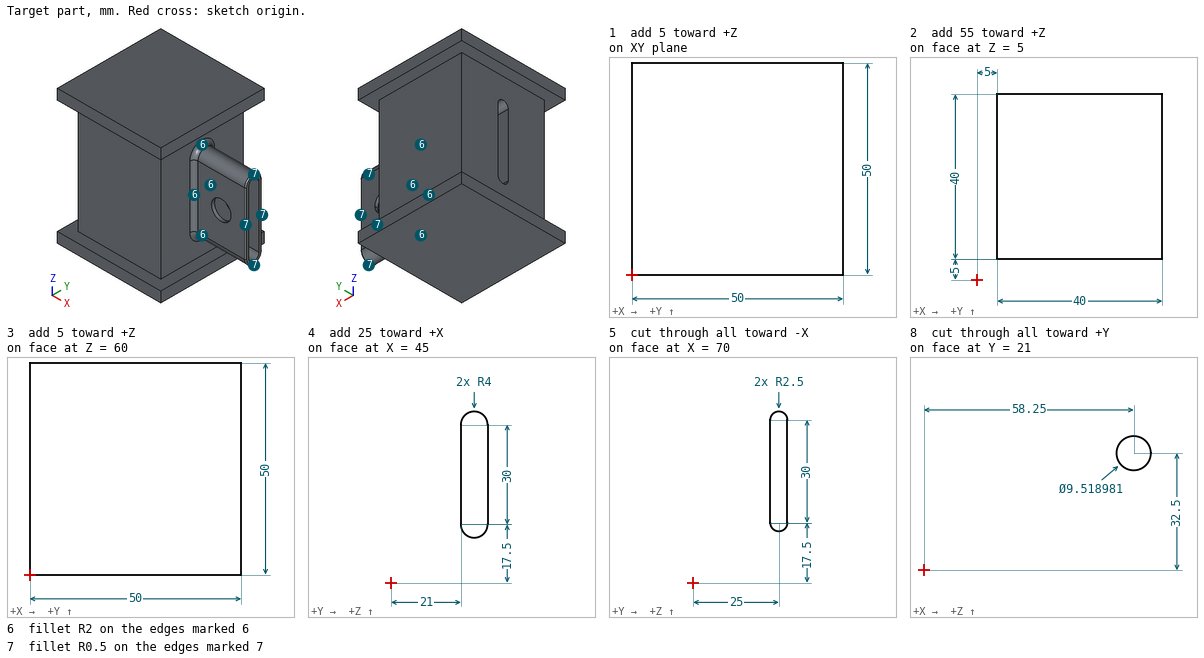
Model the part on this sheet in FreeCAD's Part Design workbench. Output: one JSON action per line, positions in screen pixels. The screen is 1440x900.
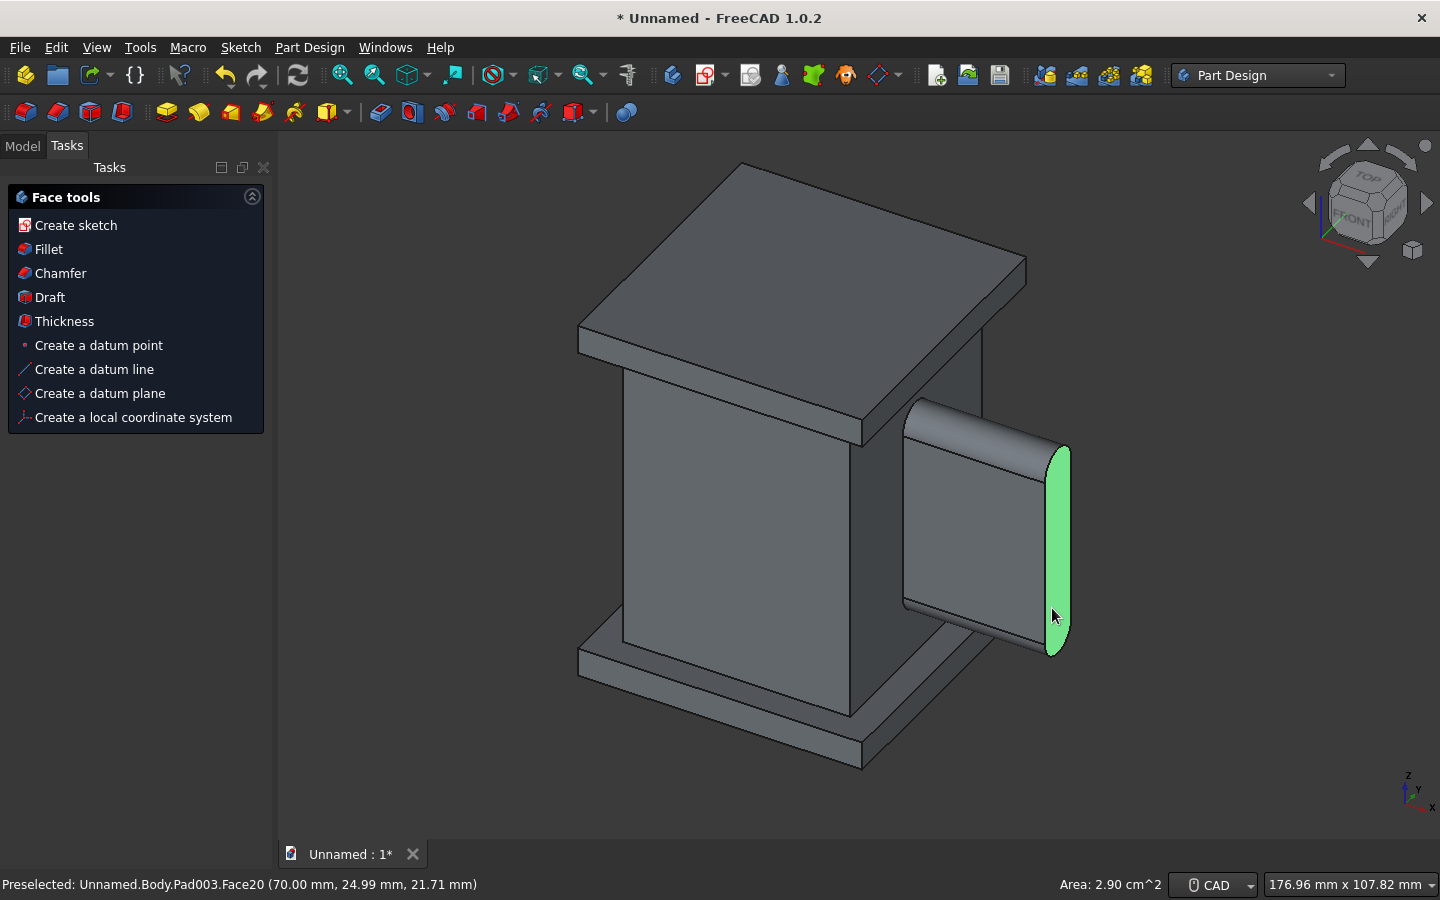
{"action": "left_click", "coordinate": [706, 76]}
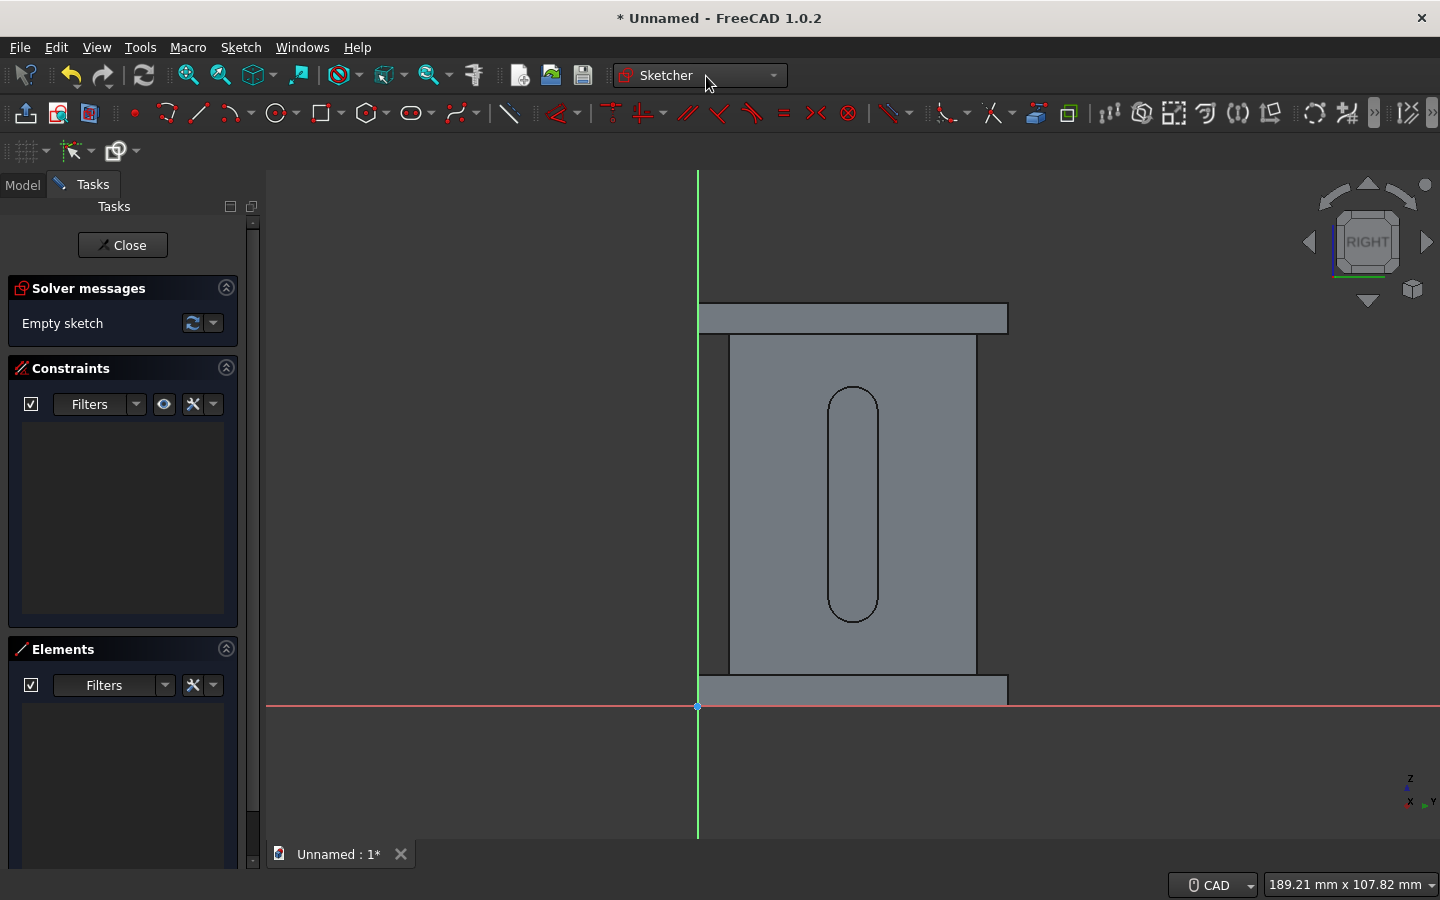
{"action": "scroll", "coordinate": [781, 646], "scroll_direction": "up", "scroll_amount": 2}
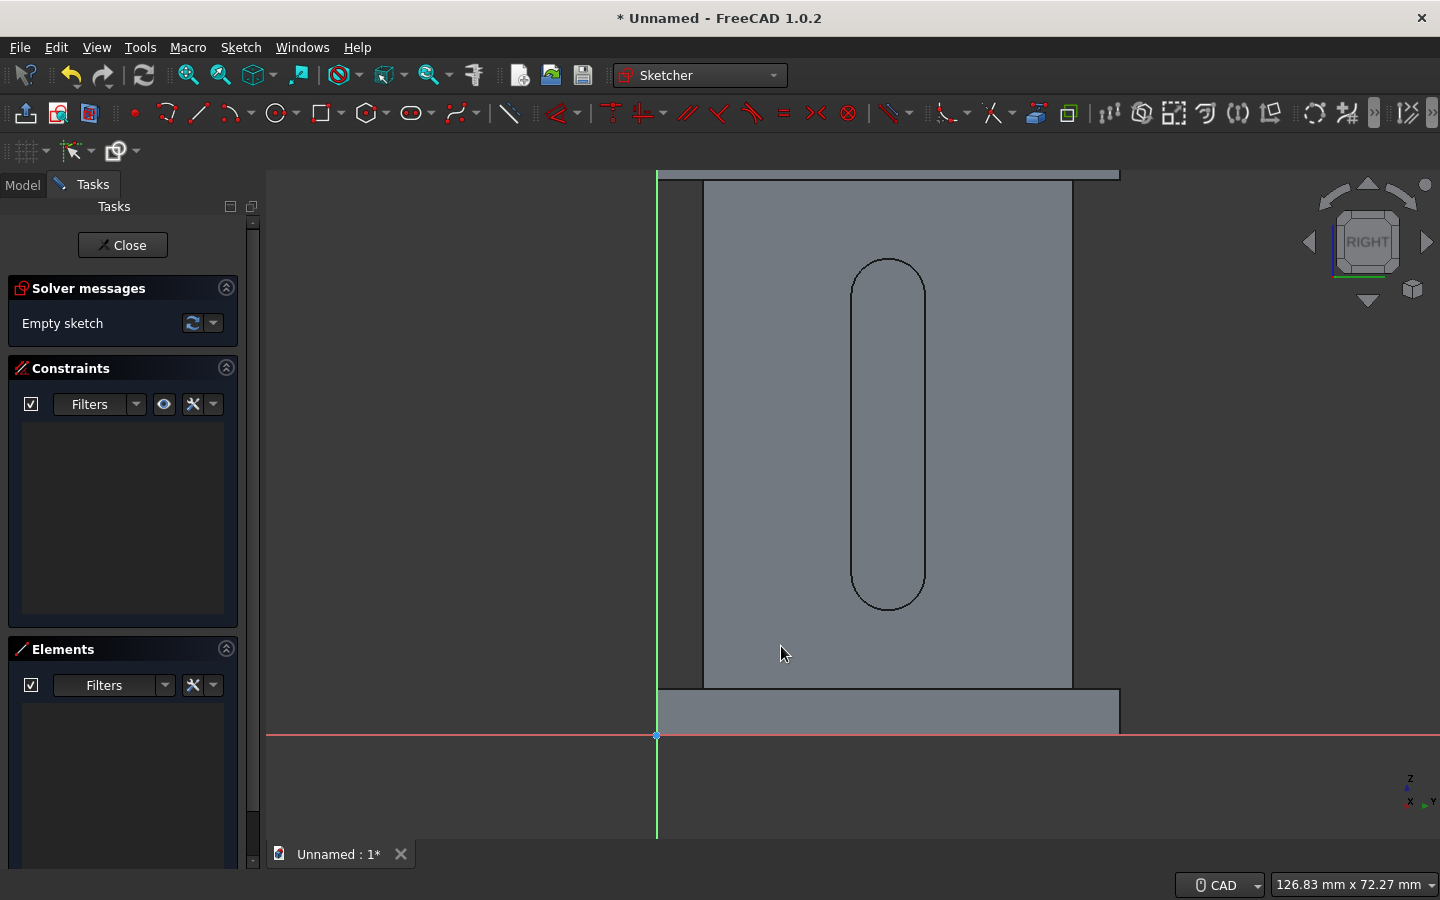
{"action": "left_click", "coordinate": [412, 114]}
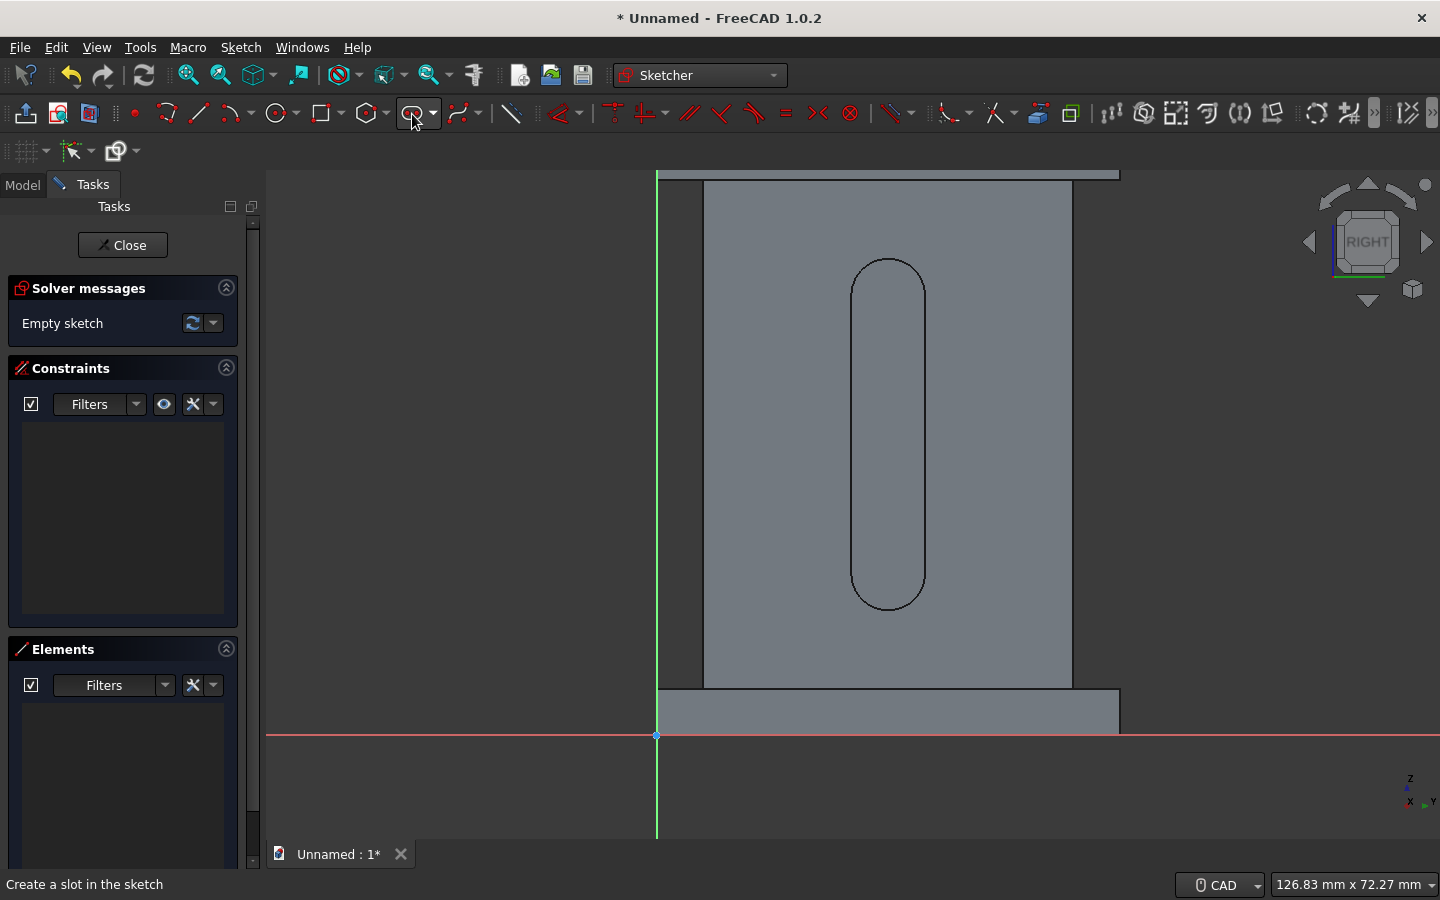
{"action": "left_click", "coordinate": [888, 573]}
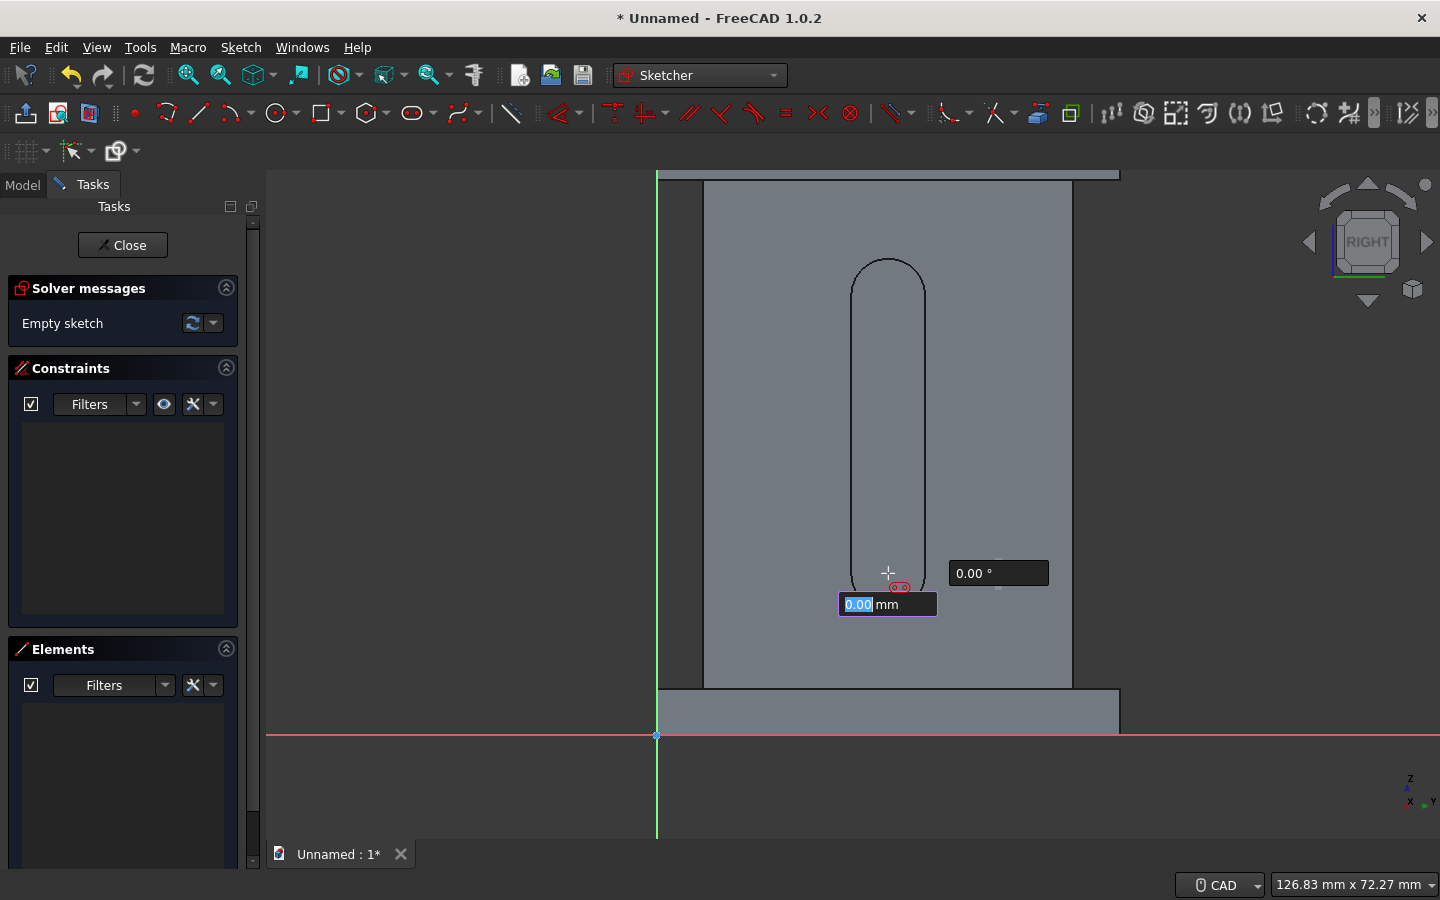
{"action": "left_click", "coordinate": [888, 296]}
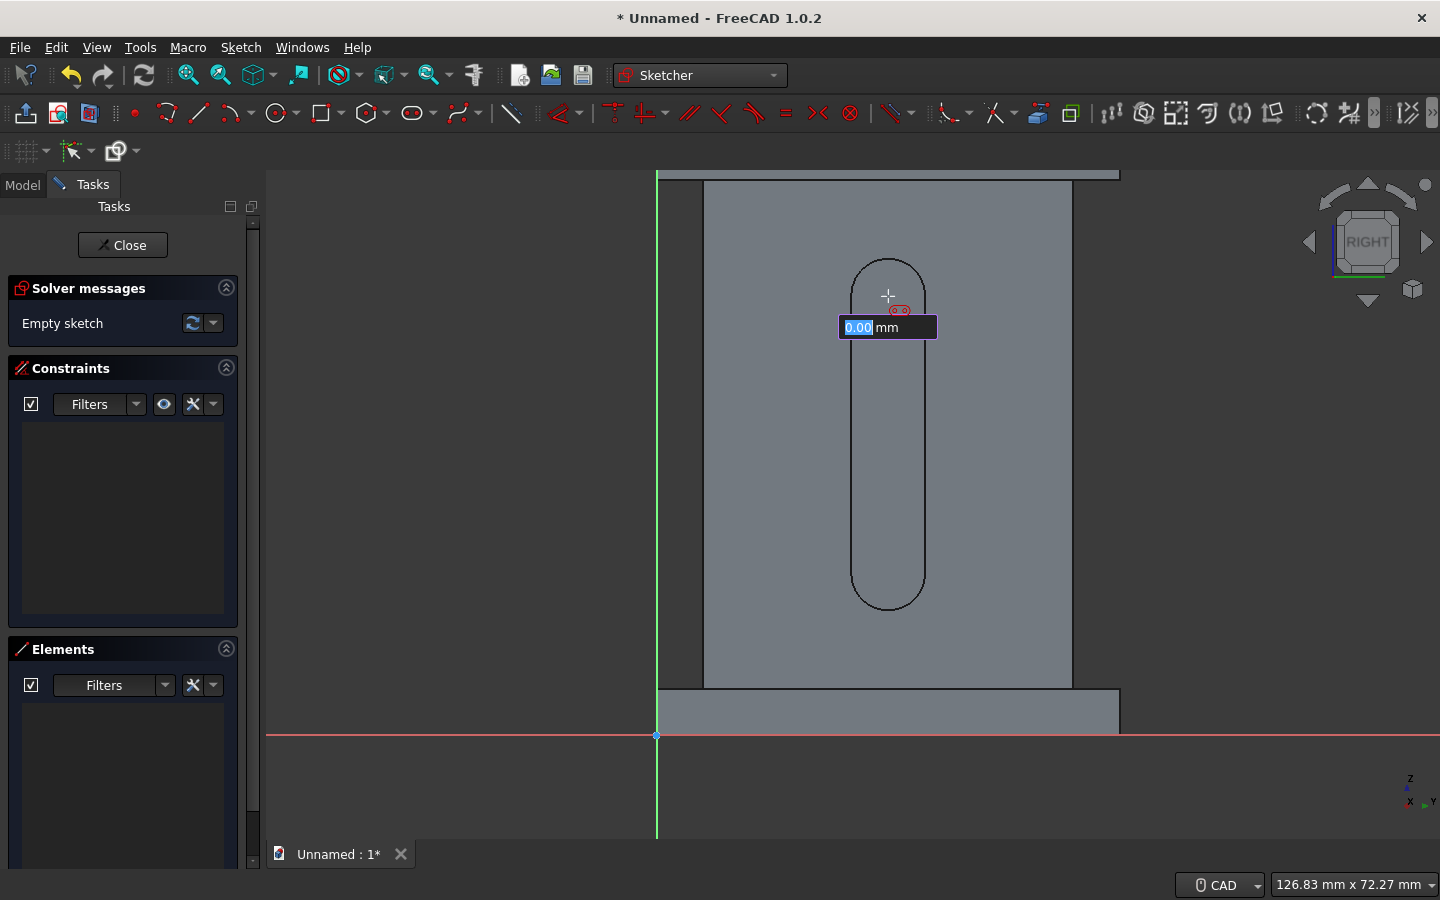
{"action": "left_click", "coordinate": [865, 435]}
{"action": "key", "text": "Escape"}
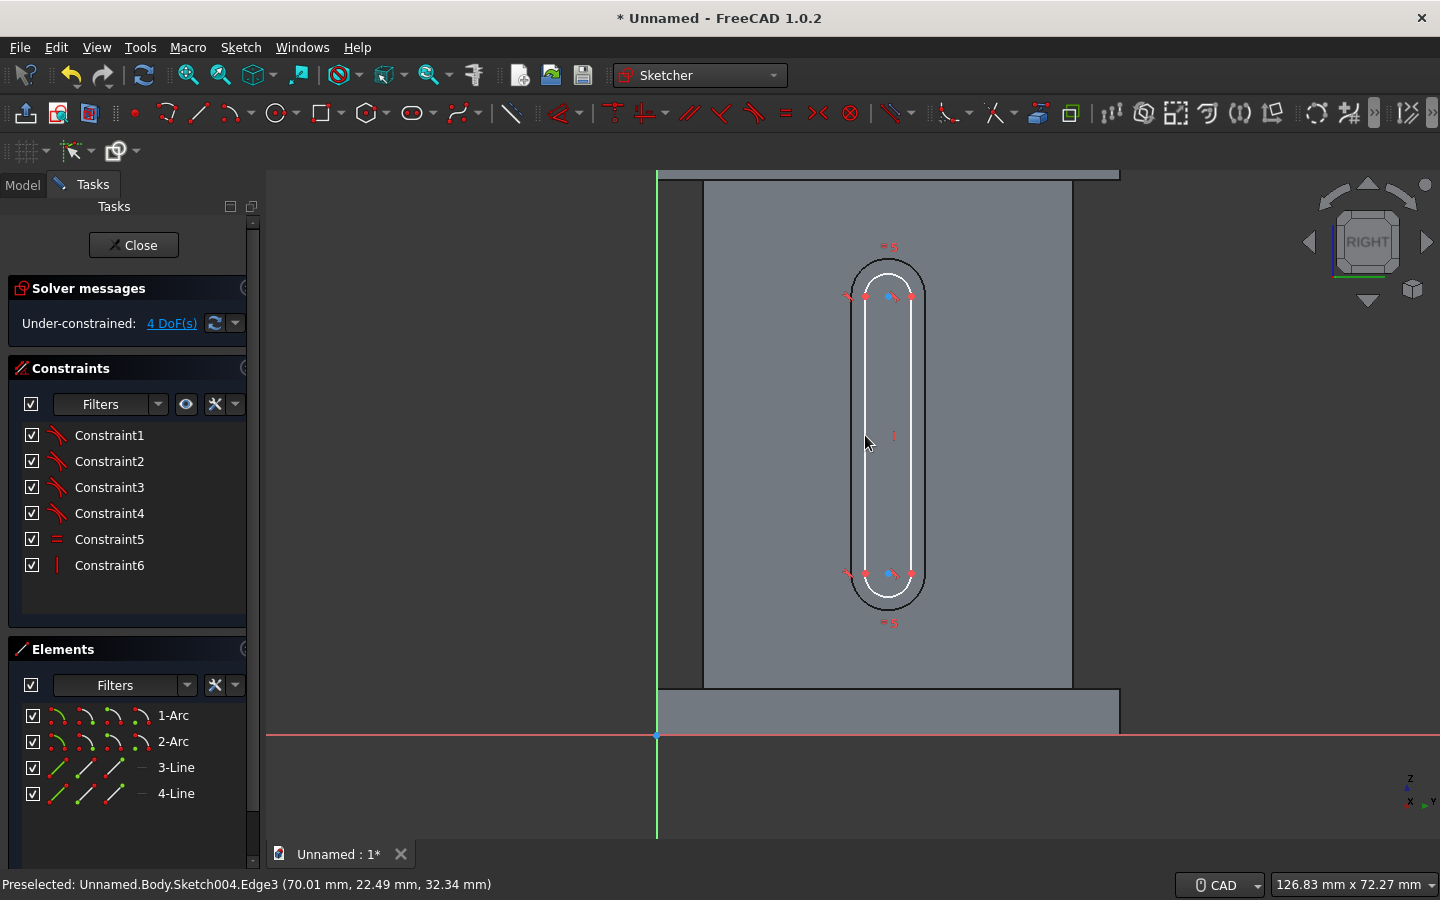
{"action": "left_click", "coordinate": [558, 114]}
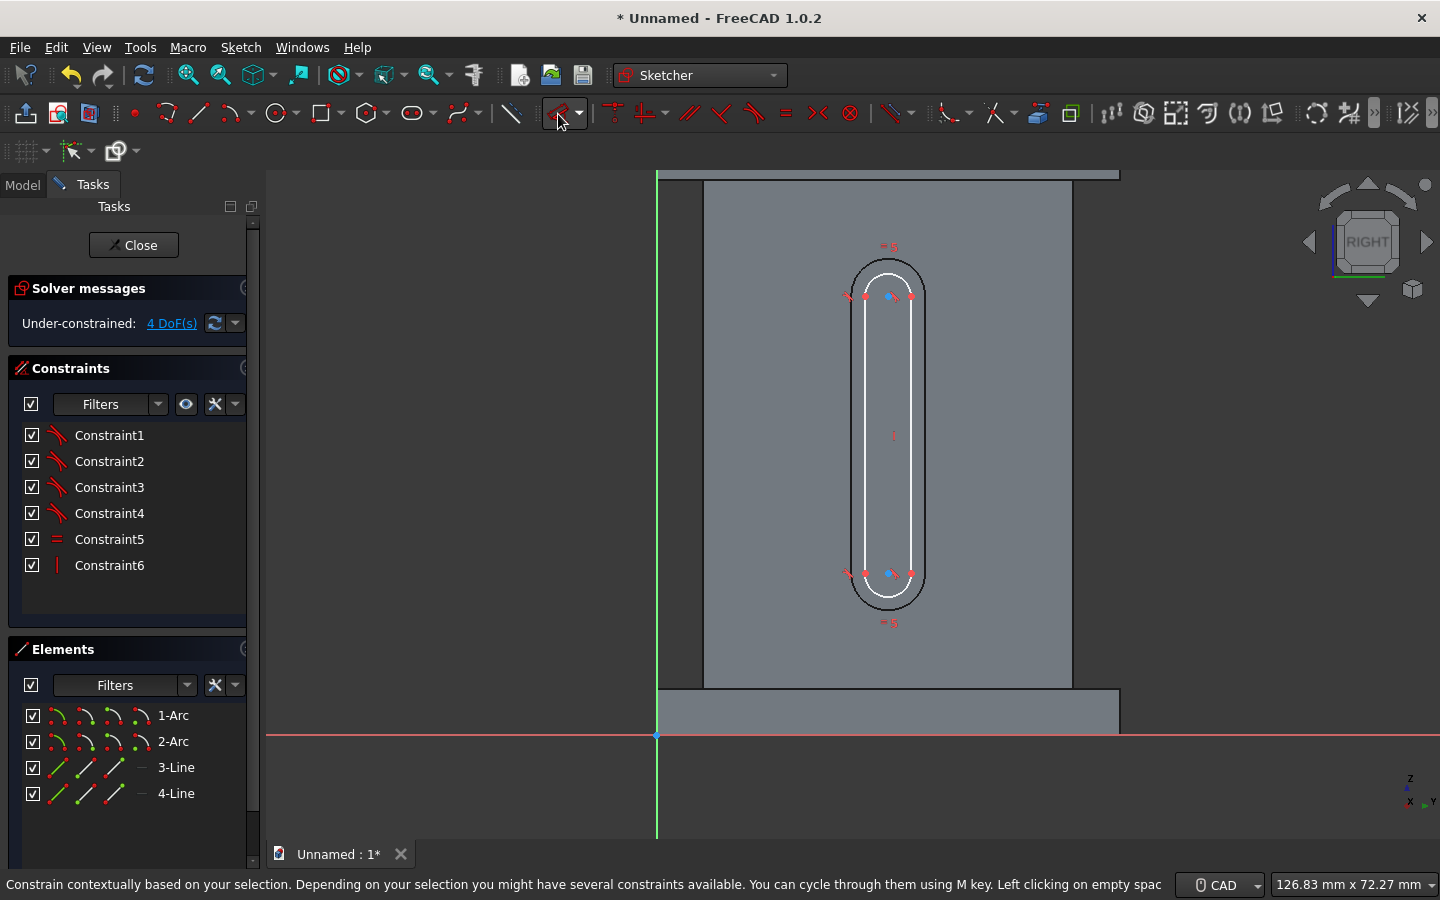
{"action": "scroll", "coordinate": [874, 593], "scroll_direction": "up", "scroll_amount": 3}